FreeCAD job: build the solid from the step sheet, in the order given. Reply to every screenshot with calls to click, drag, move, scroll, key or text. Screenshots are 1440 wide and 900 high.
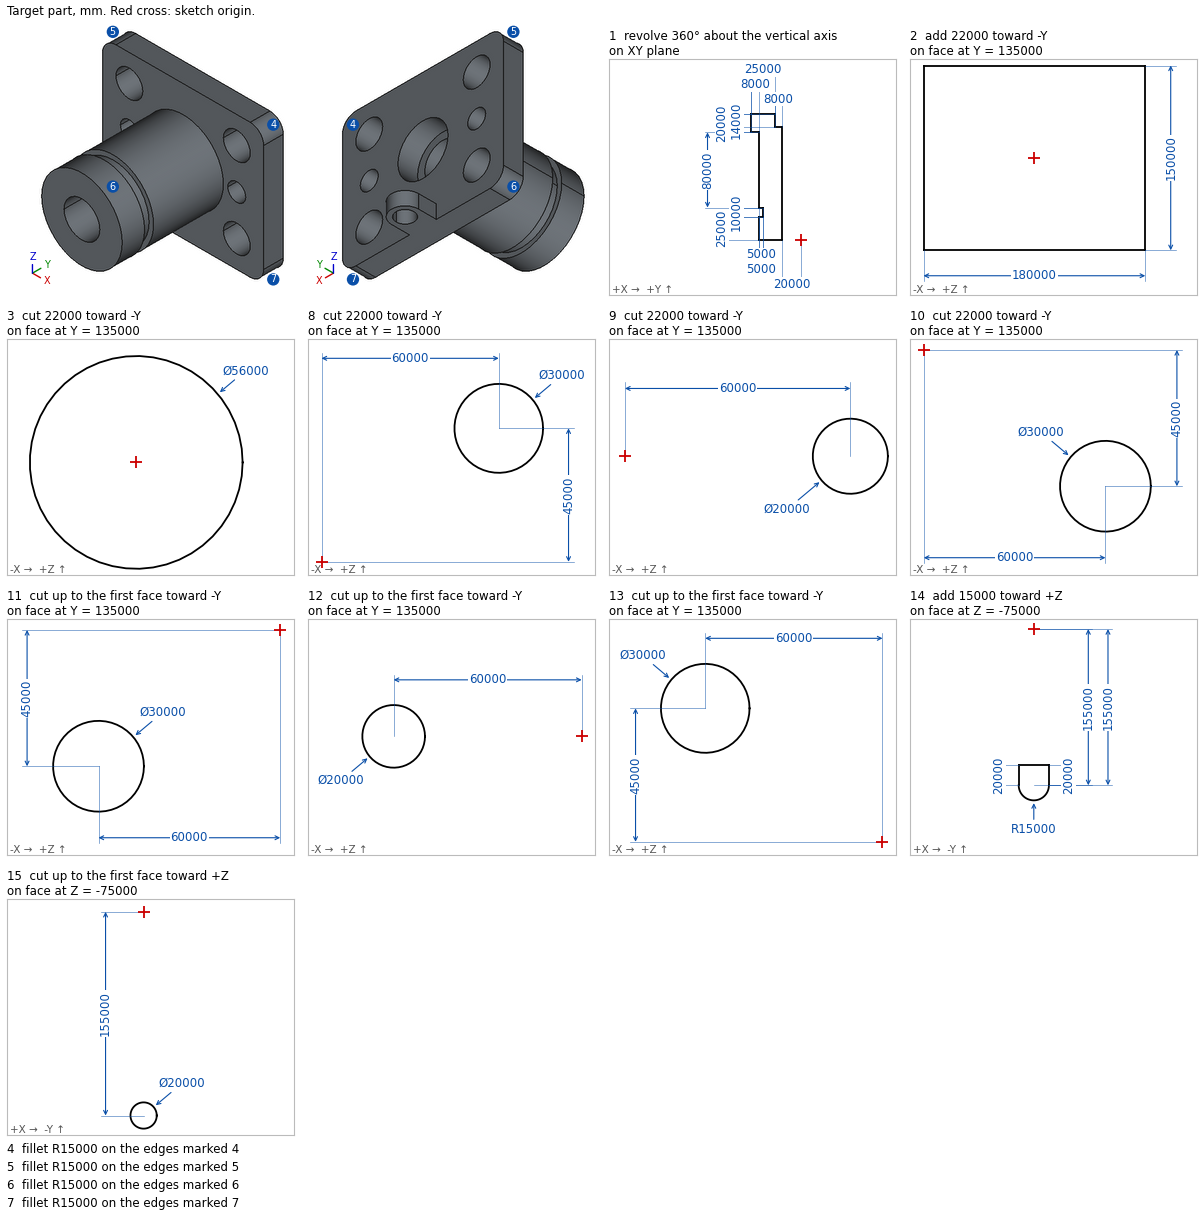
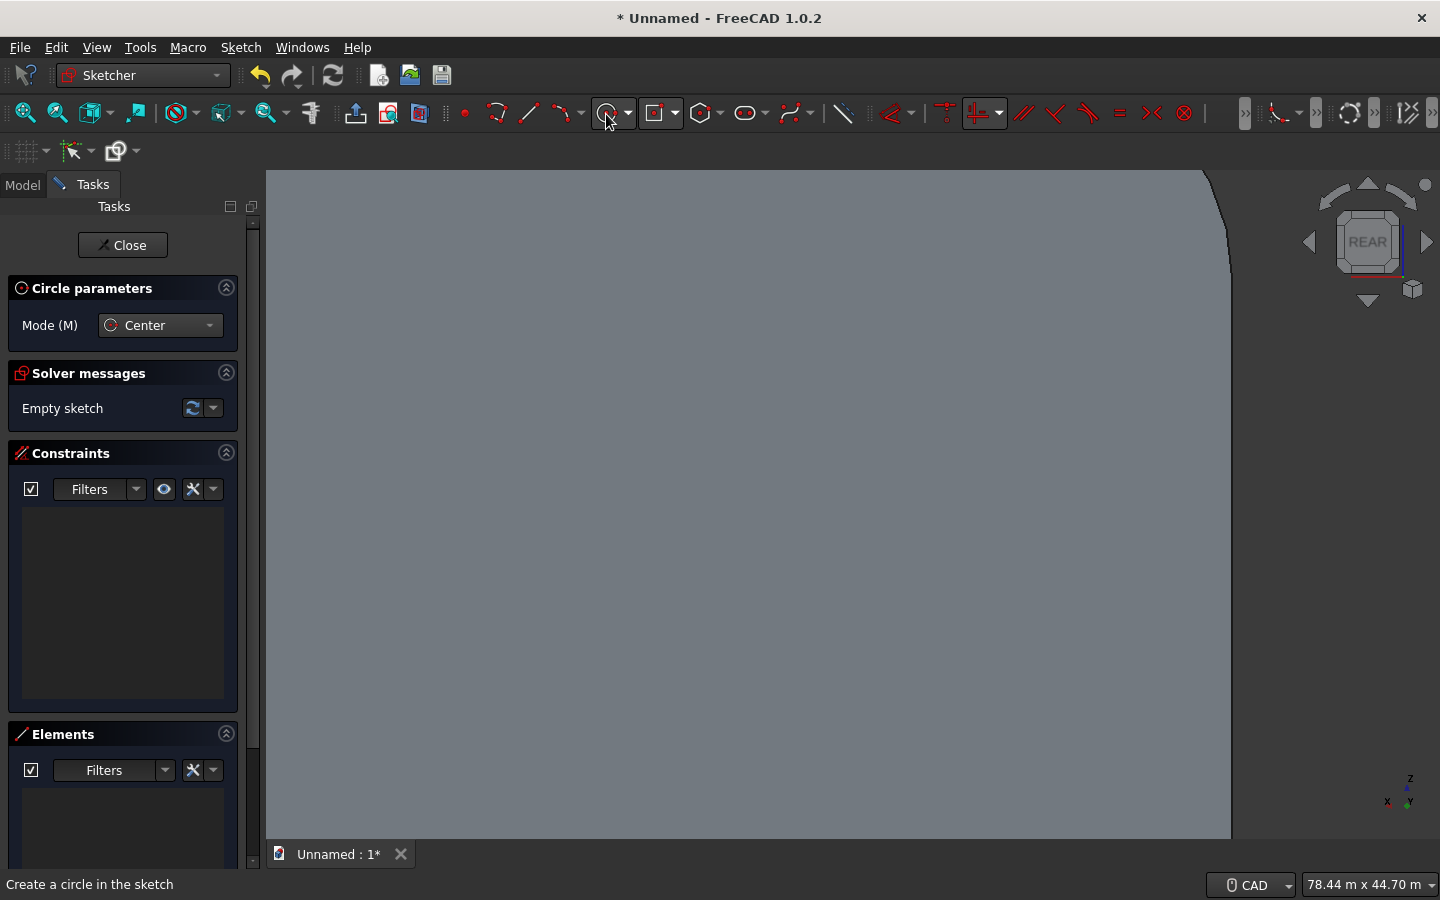
click(783, 504)
click(942, 345)
key(Escape)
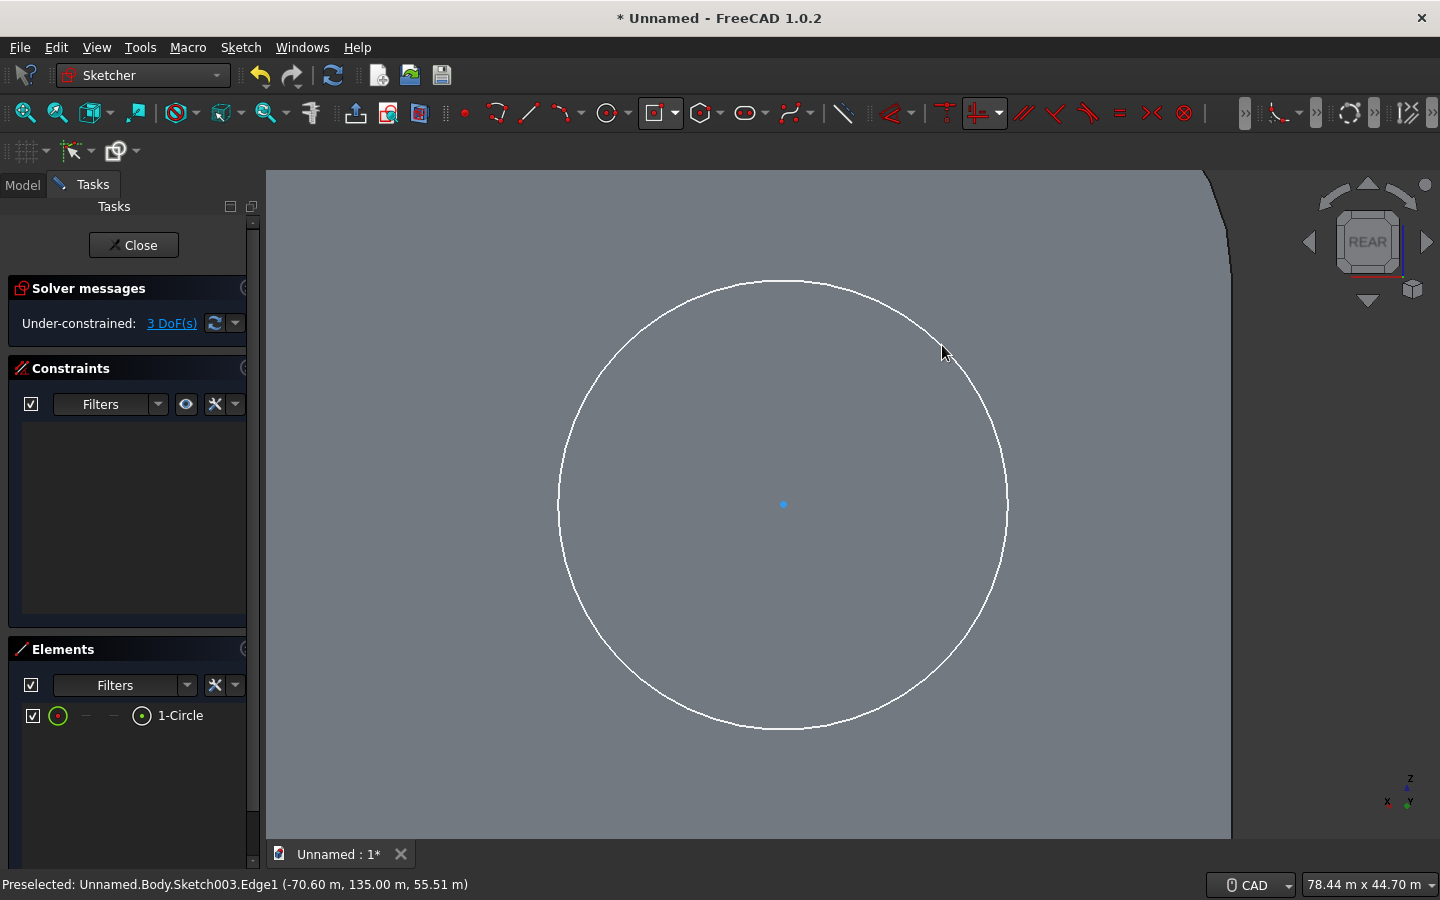
click(890, 114)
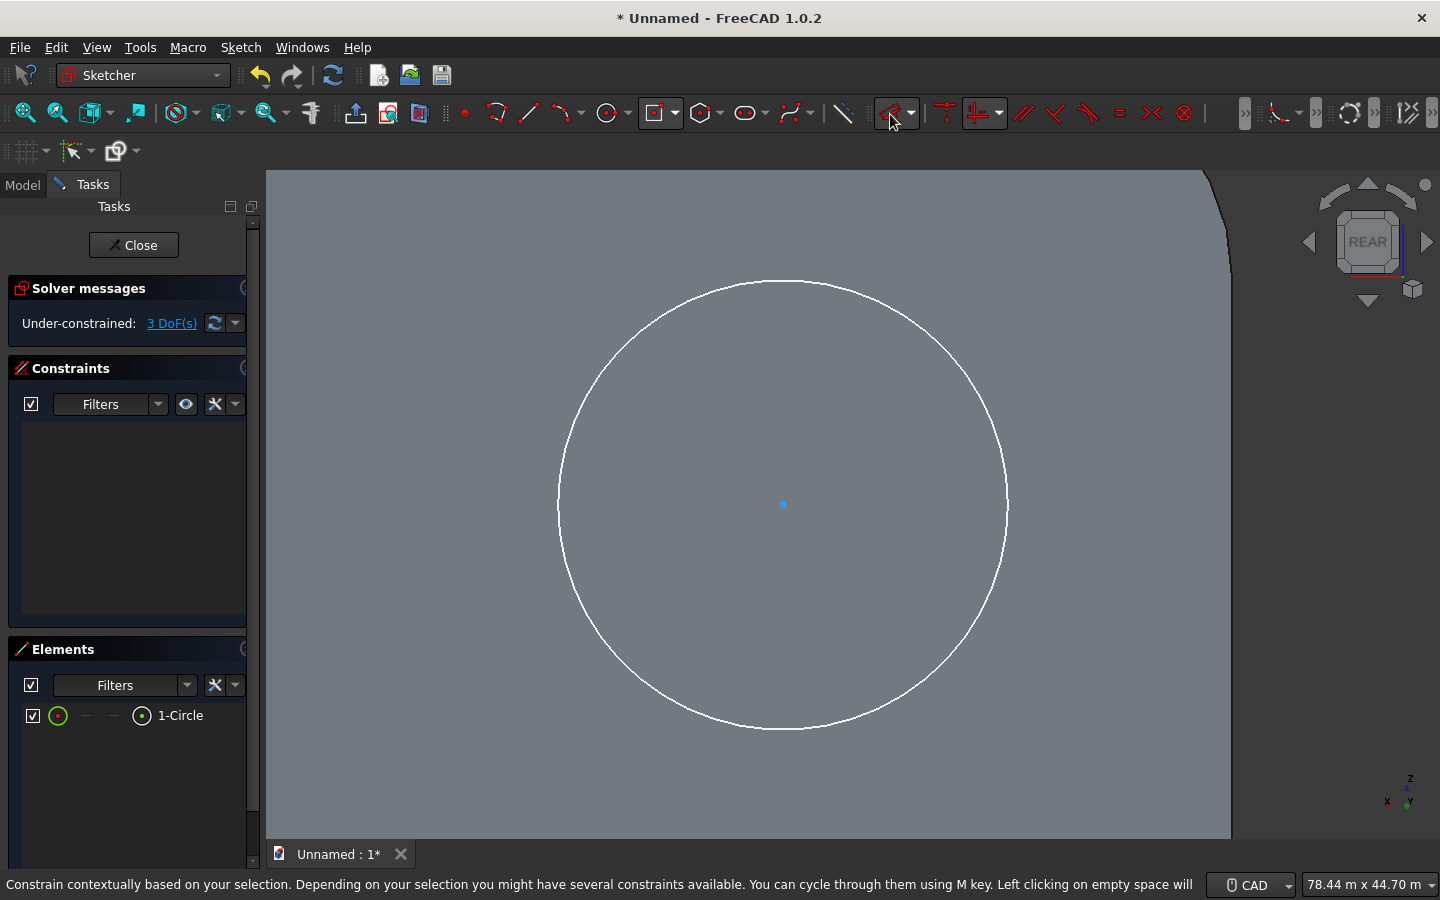
click(942, 346)
click(965, 323)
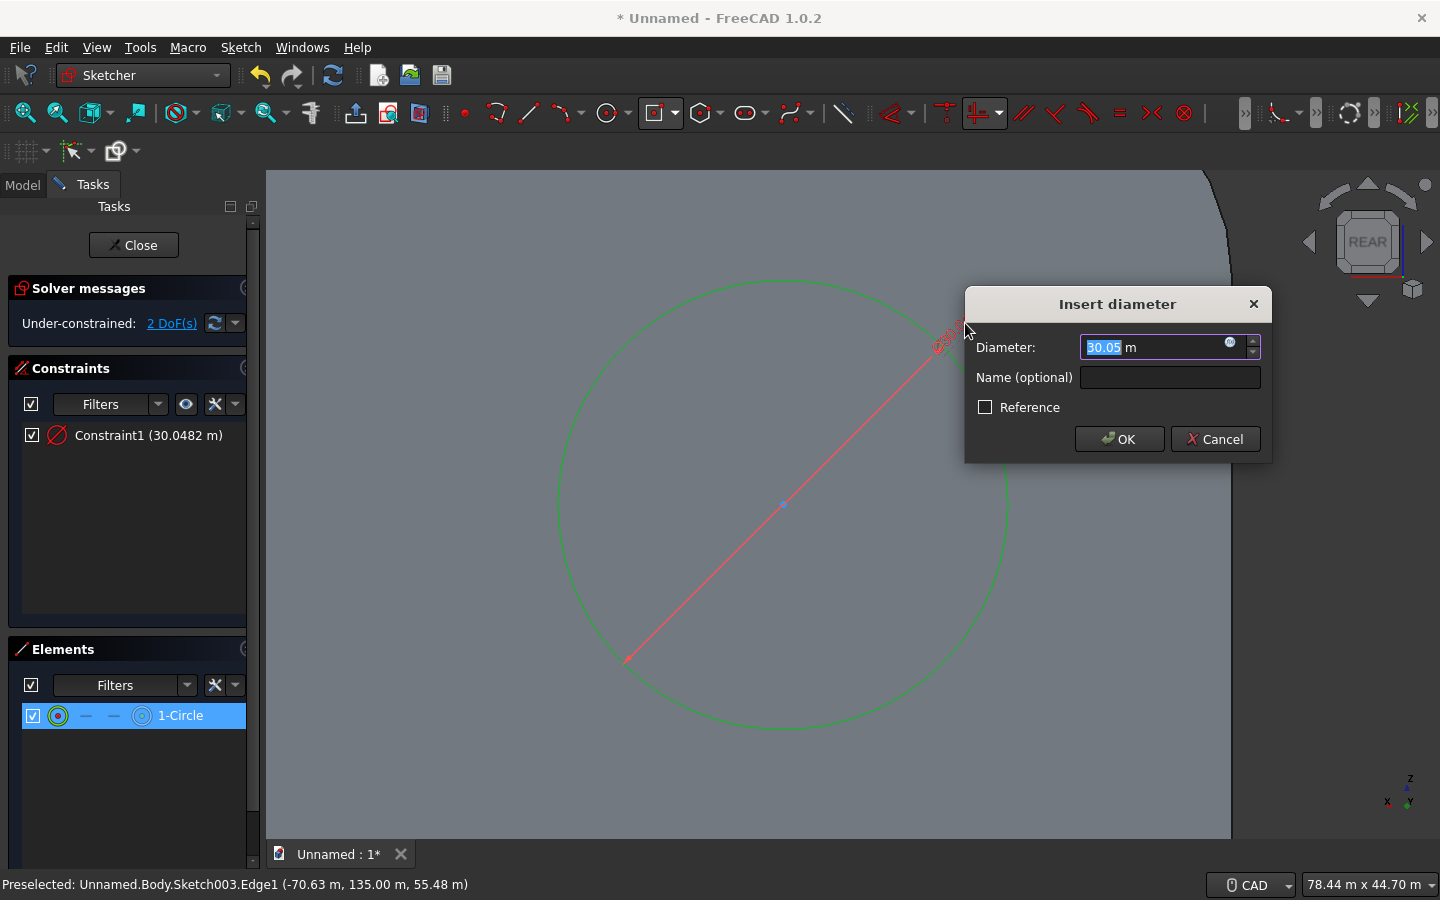
key(ctrl+a)
text(30000 mm)
key(Return)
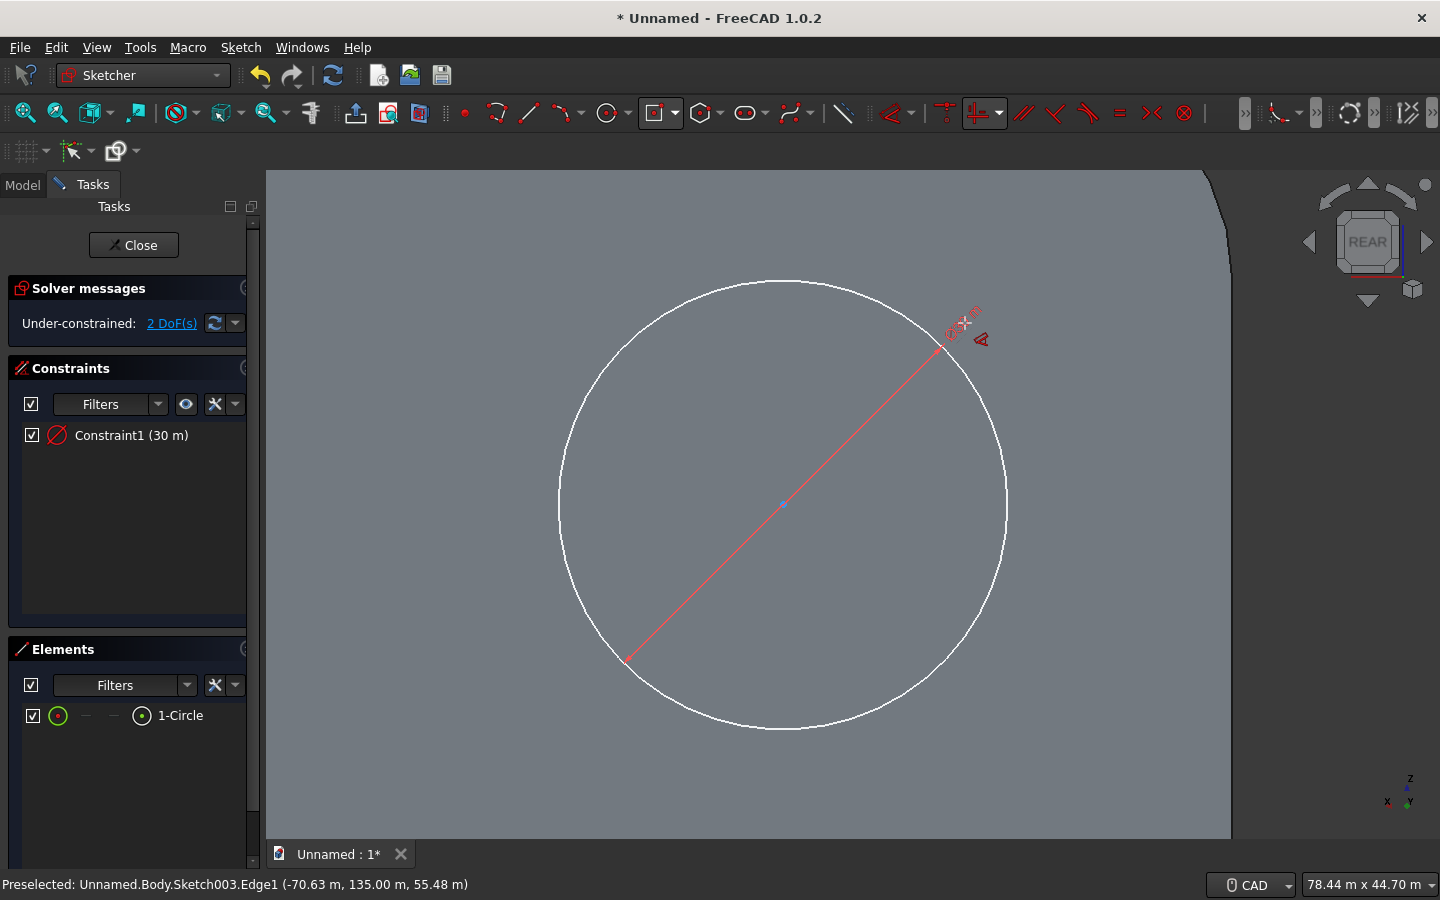
click(783, 505)
click(538, 471)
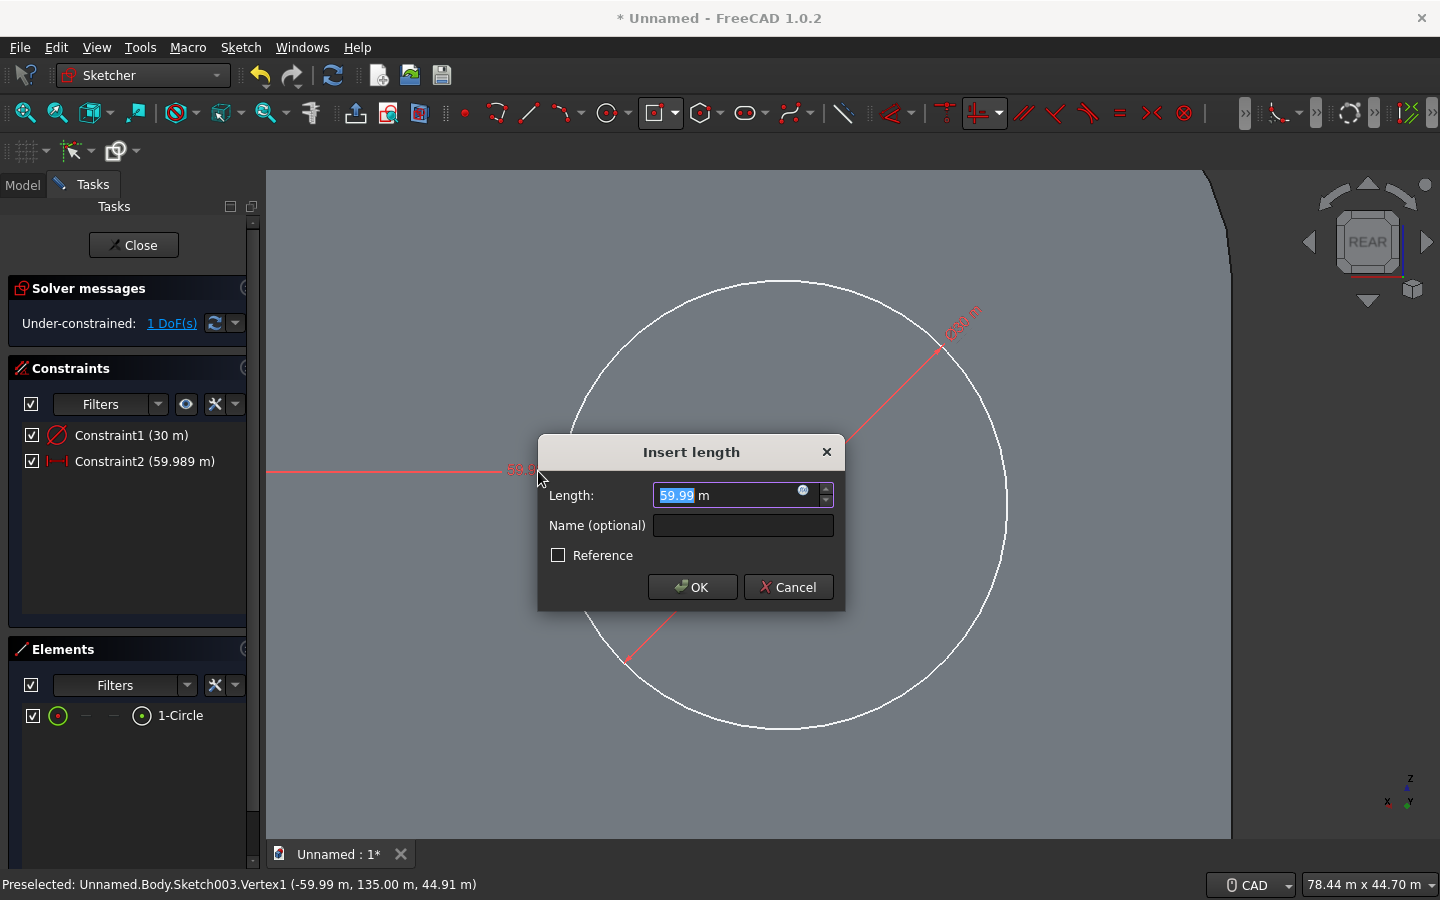
key(ctrl+a)
text(60000 mm)
key(Return)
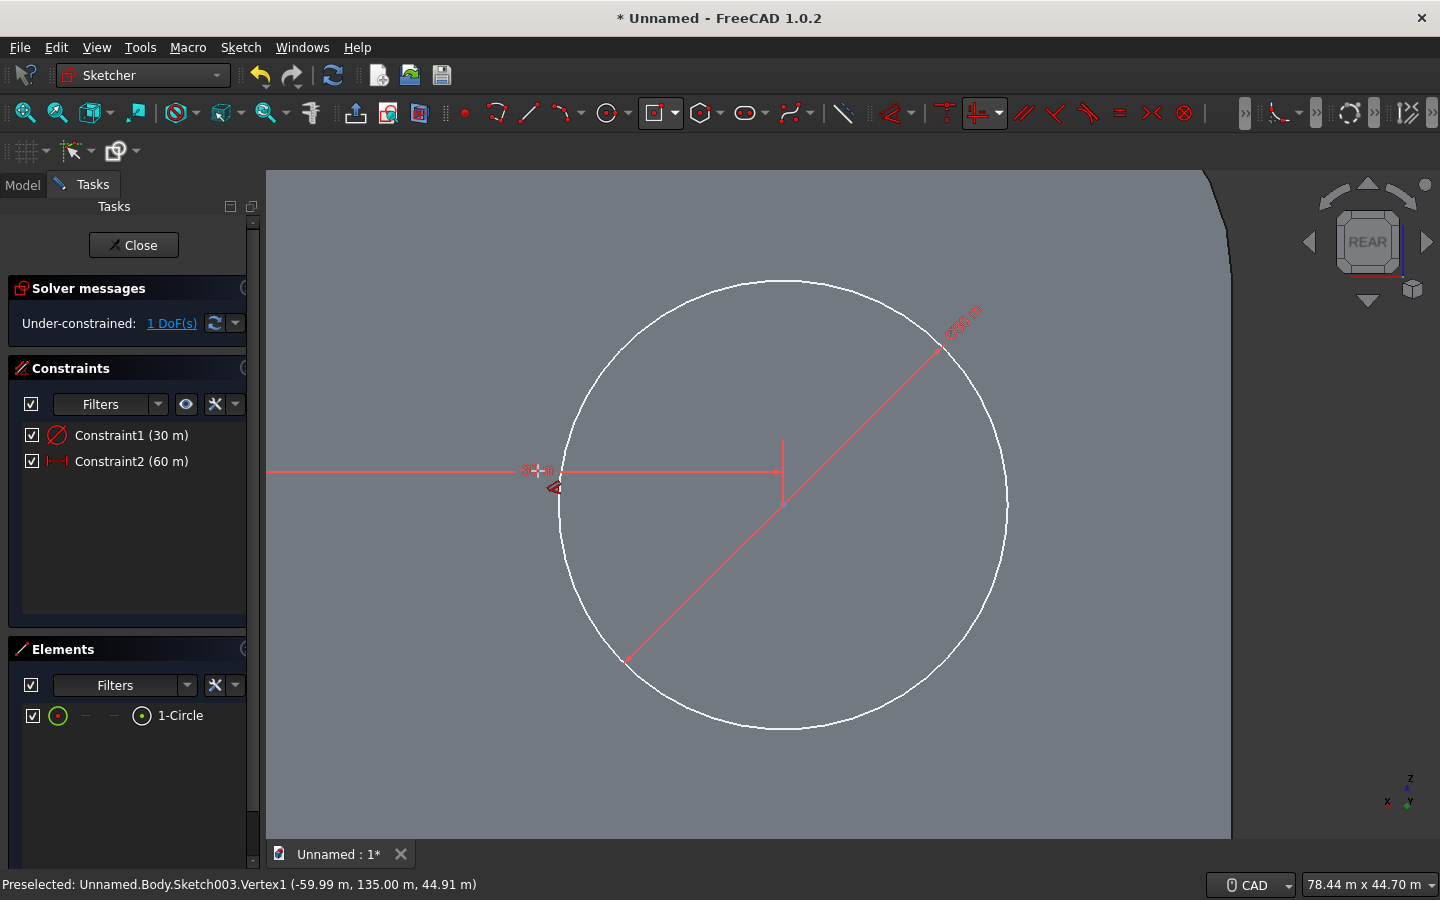
click(783, 505)
click(817, 658)